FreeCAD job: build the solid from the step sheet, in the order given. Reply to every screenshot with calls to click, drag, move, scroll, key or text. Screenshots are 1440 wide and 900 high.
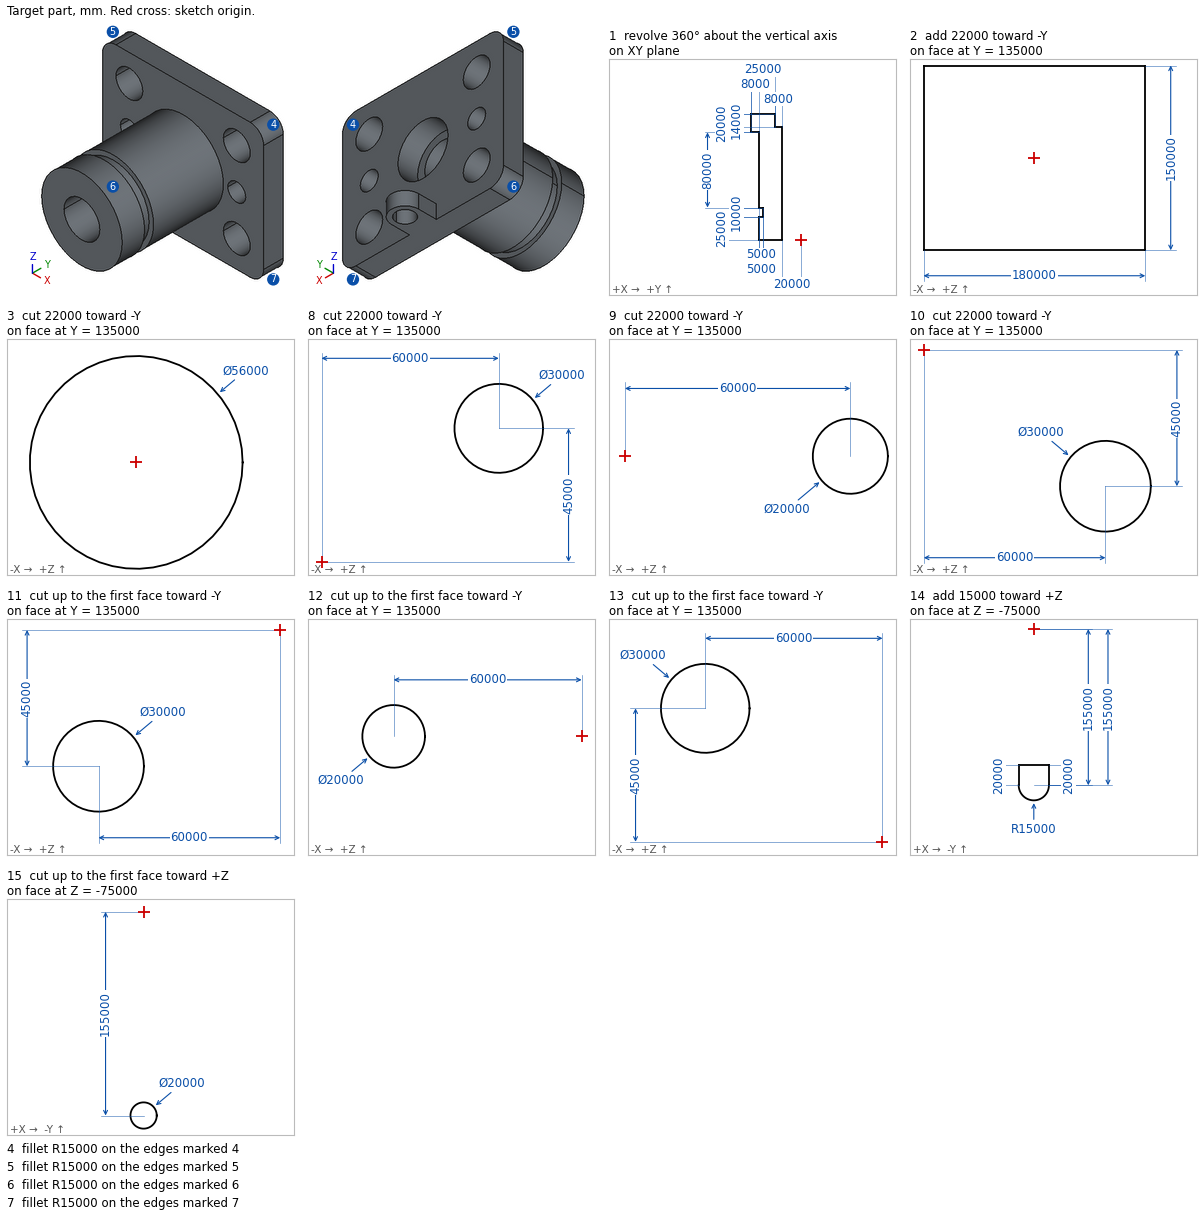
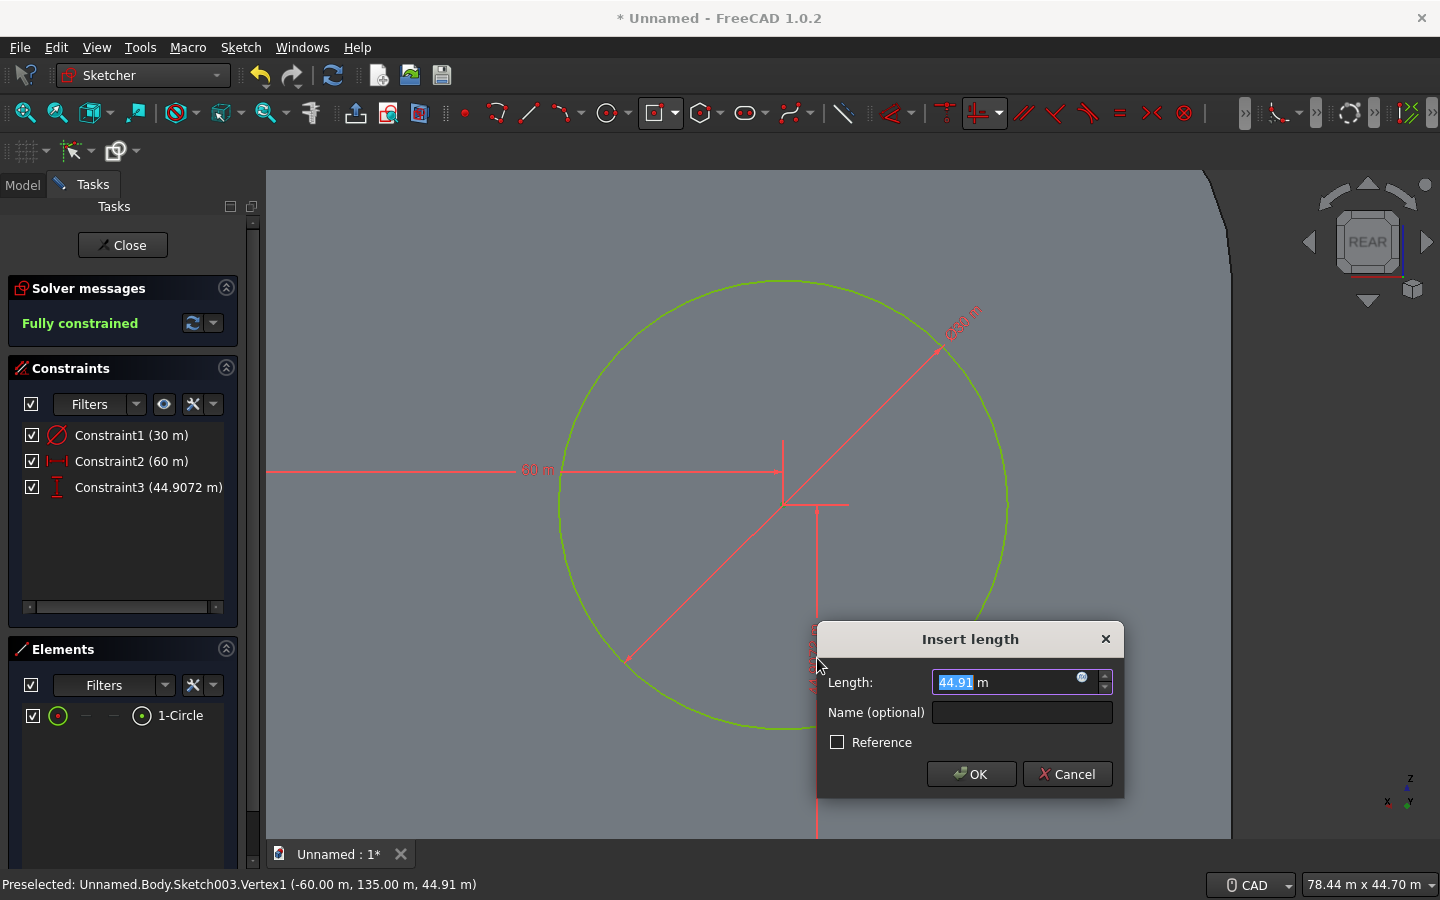
key(ctrl+a)
text(45000 mm)
key(Return)
key(Escape)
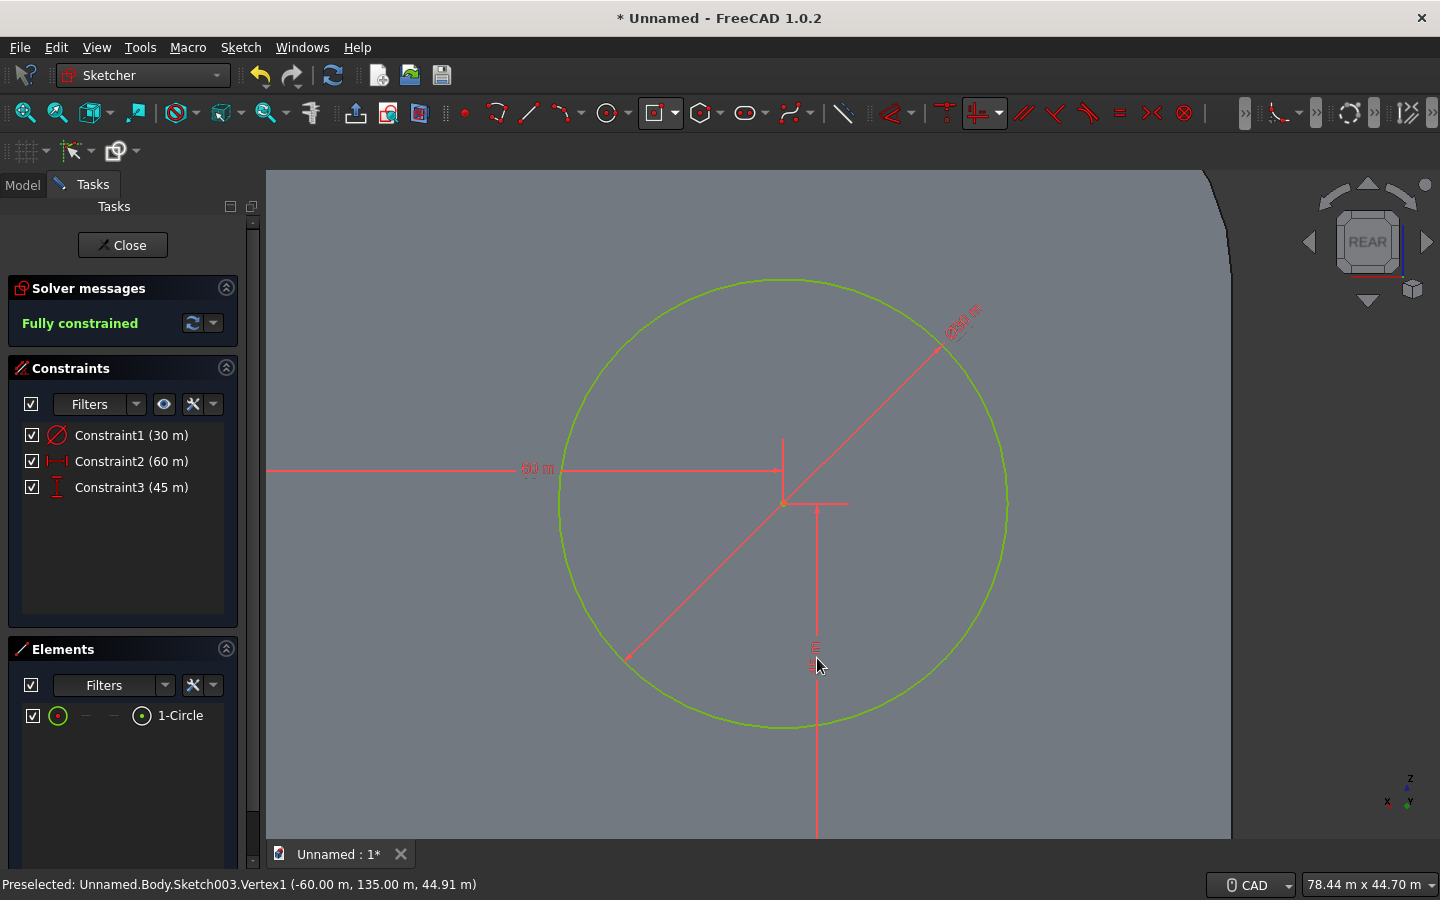
click(123, 245)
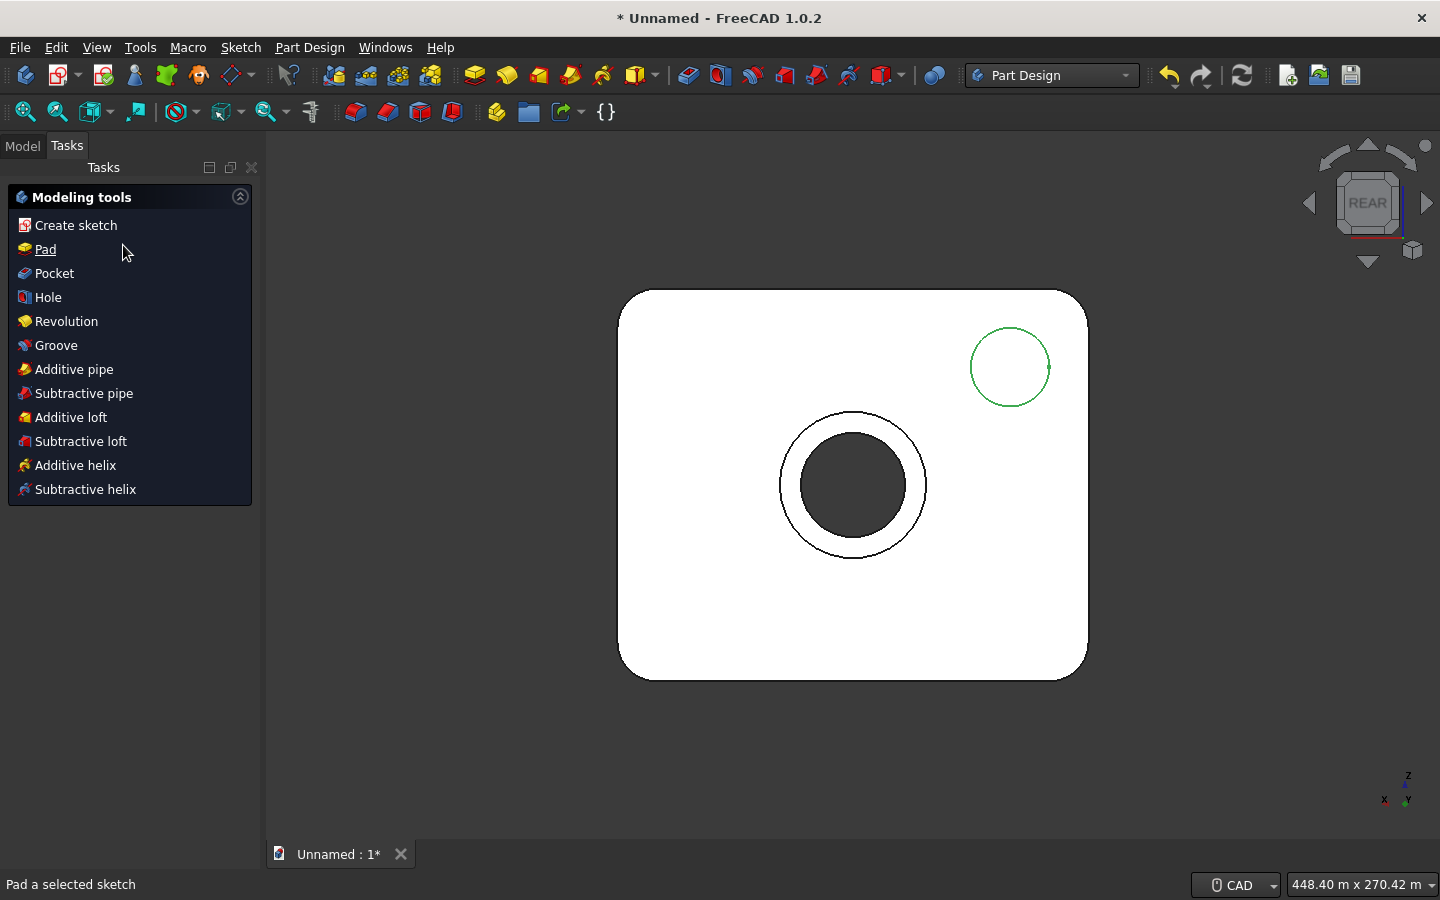
click(690, 76)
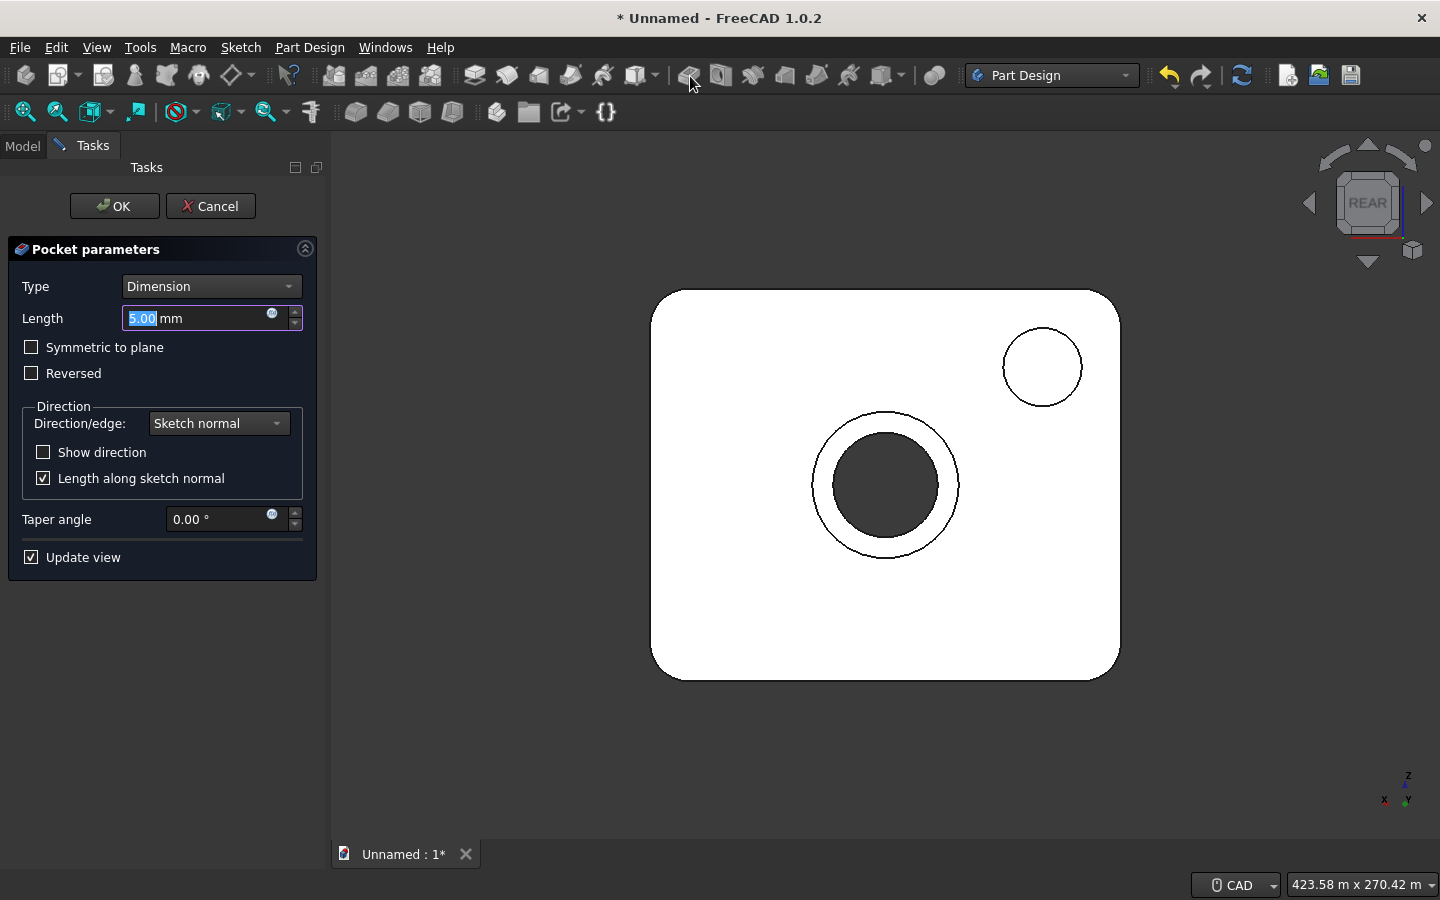
text(22000)
key(Tab)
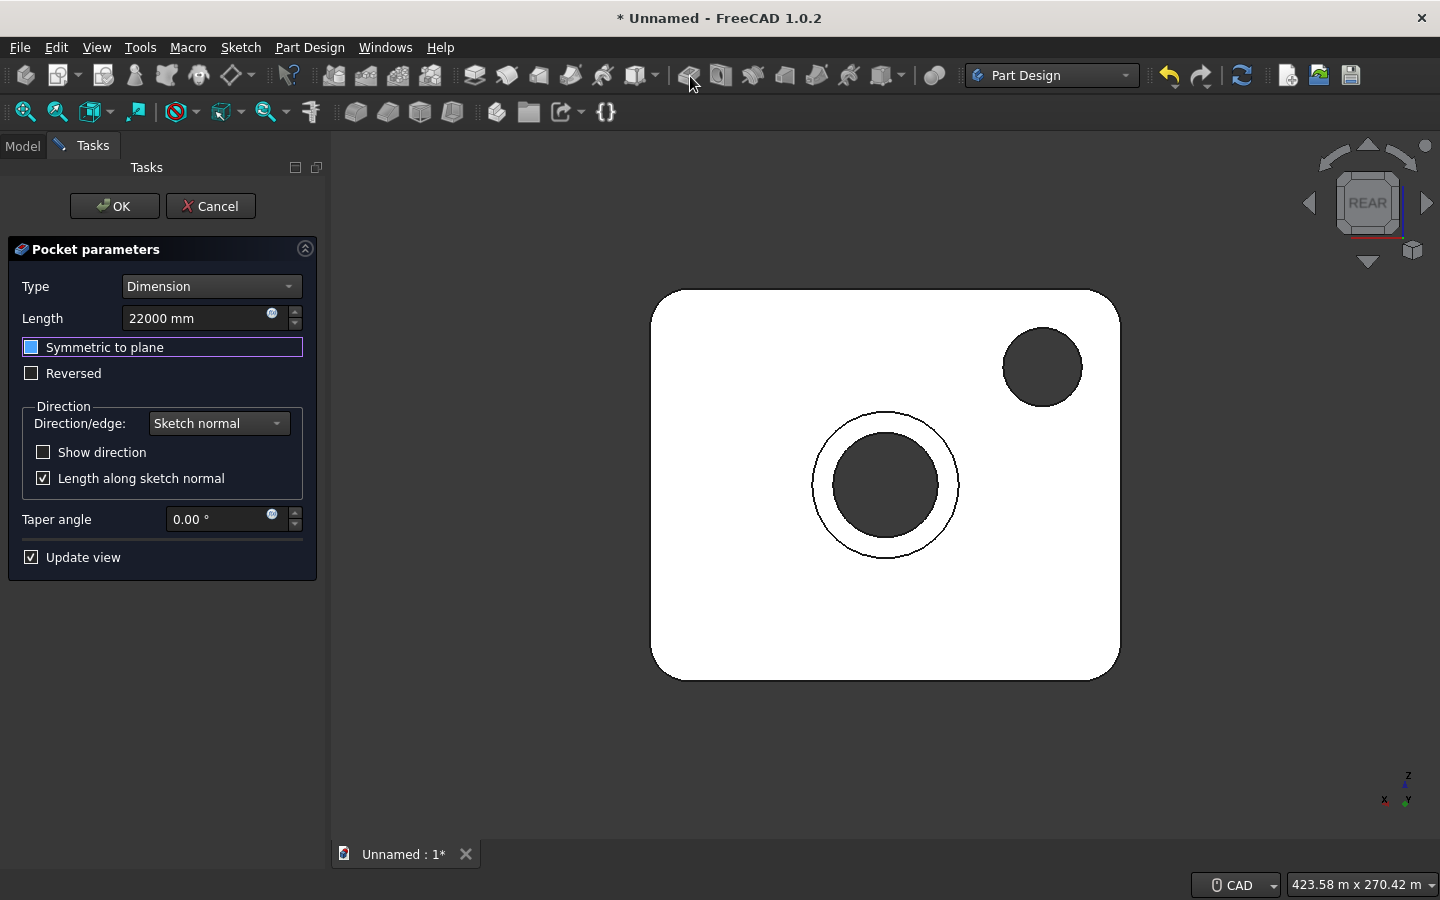
click(115, 206)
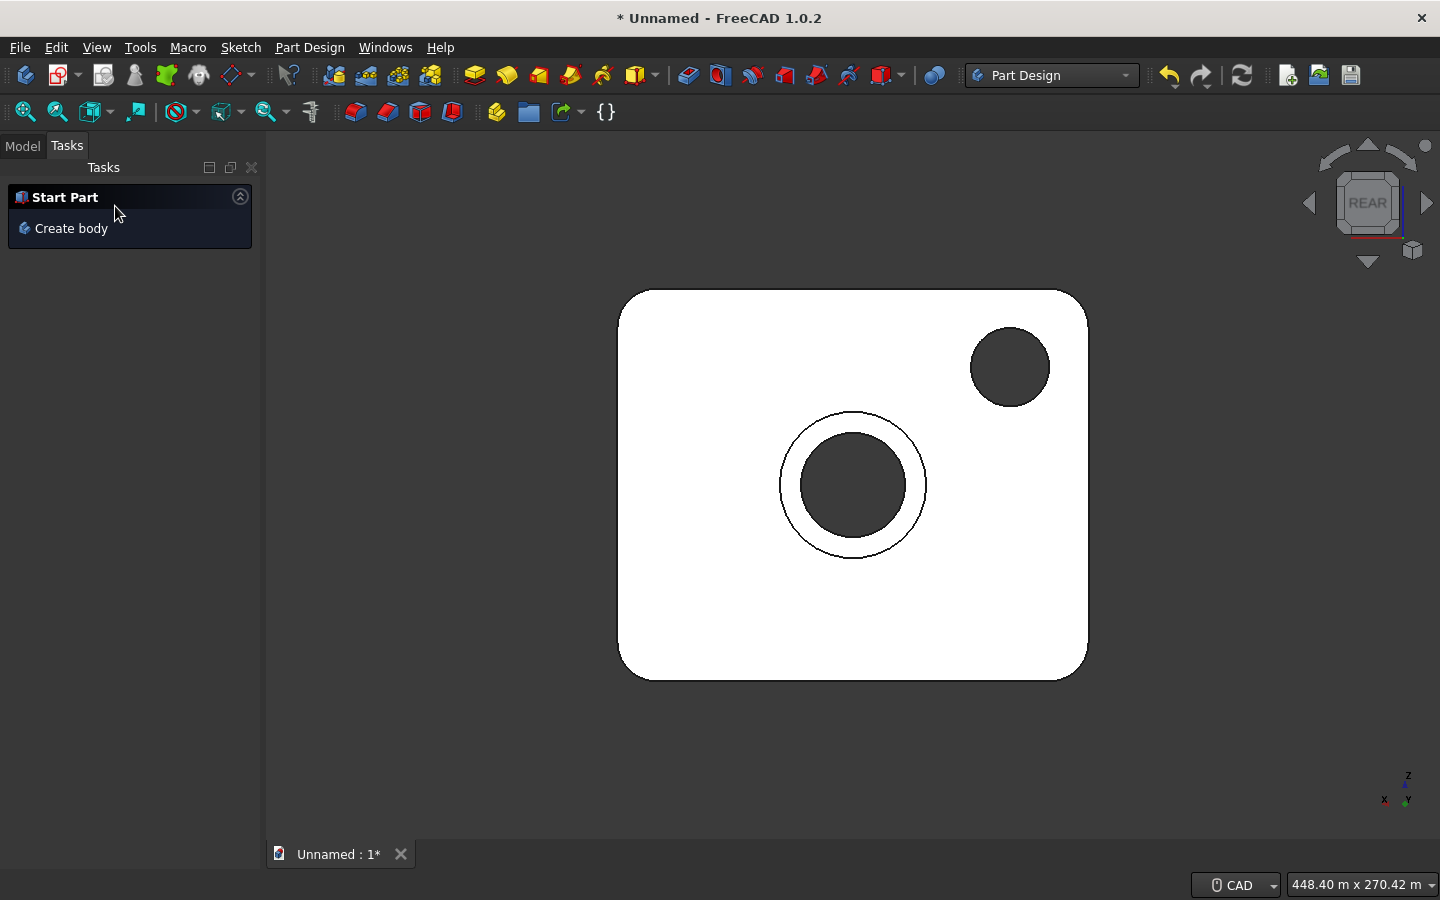
click(718, 372)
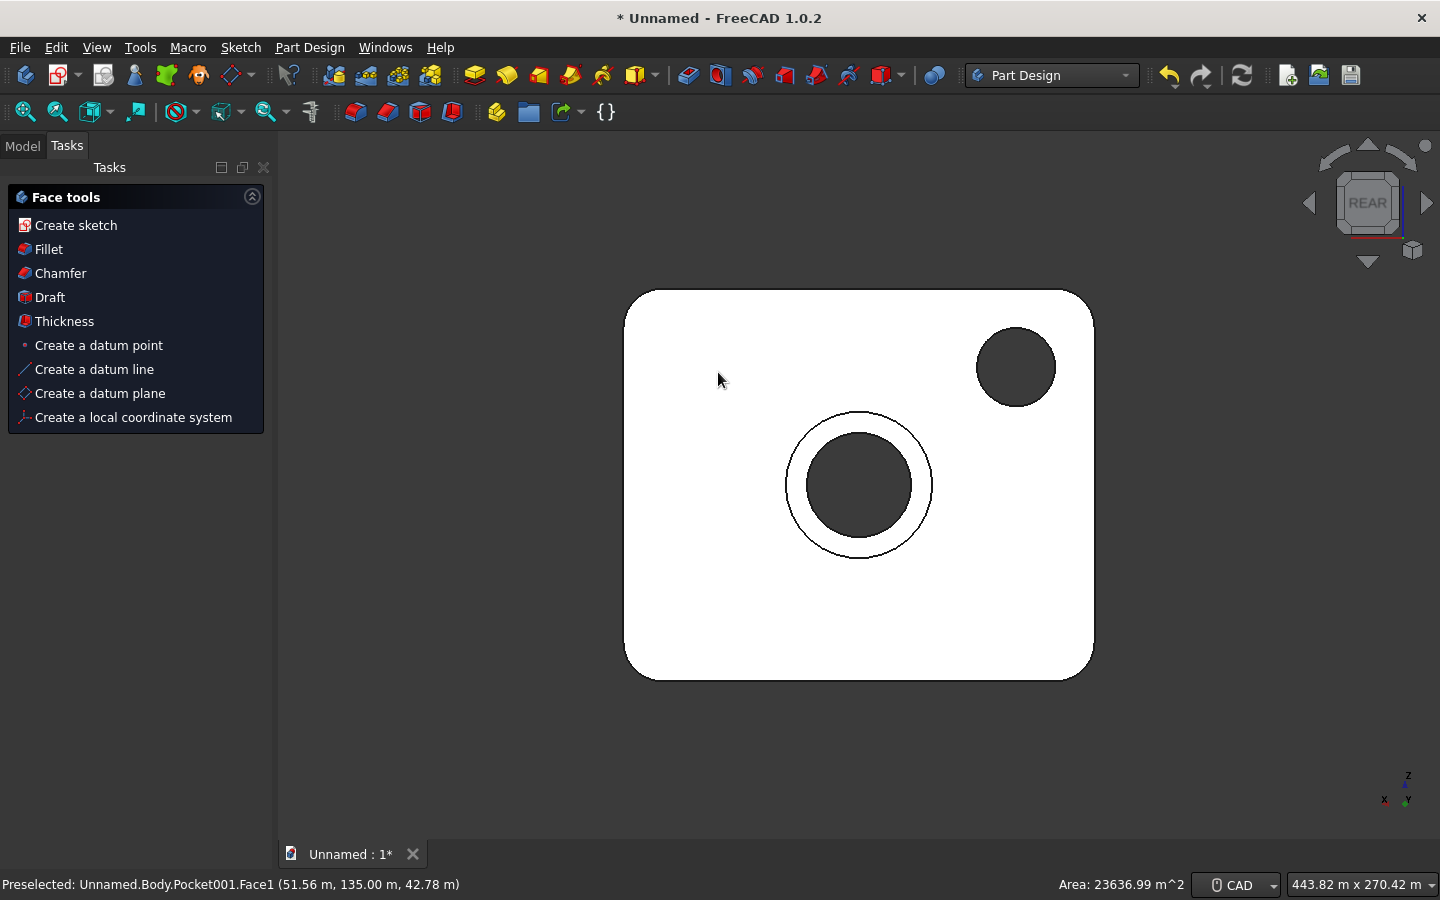
click(58, 76)